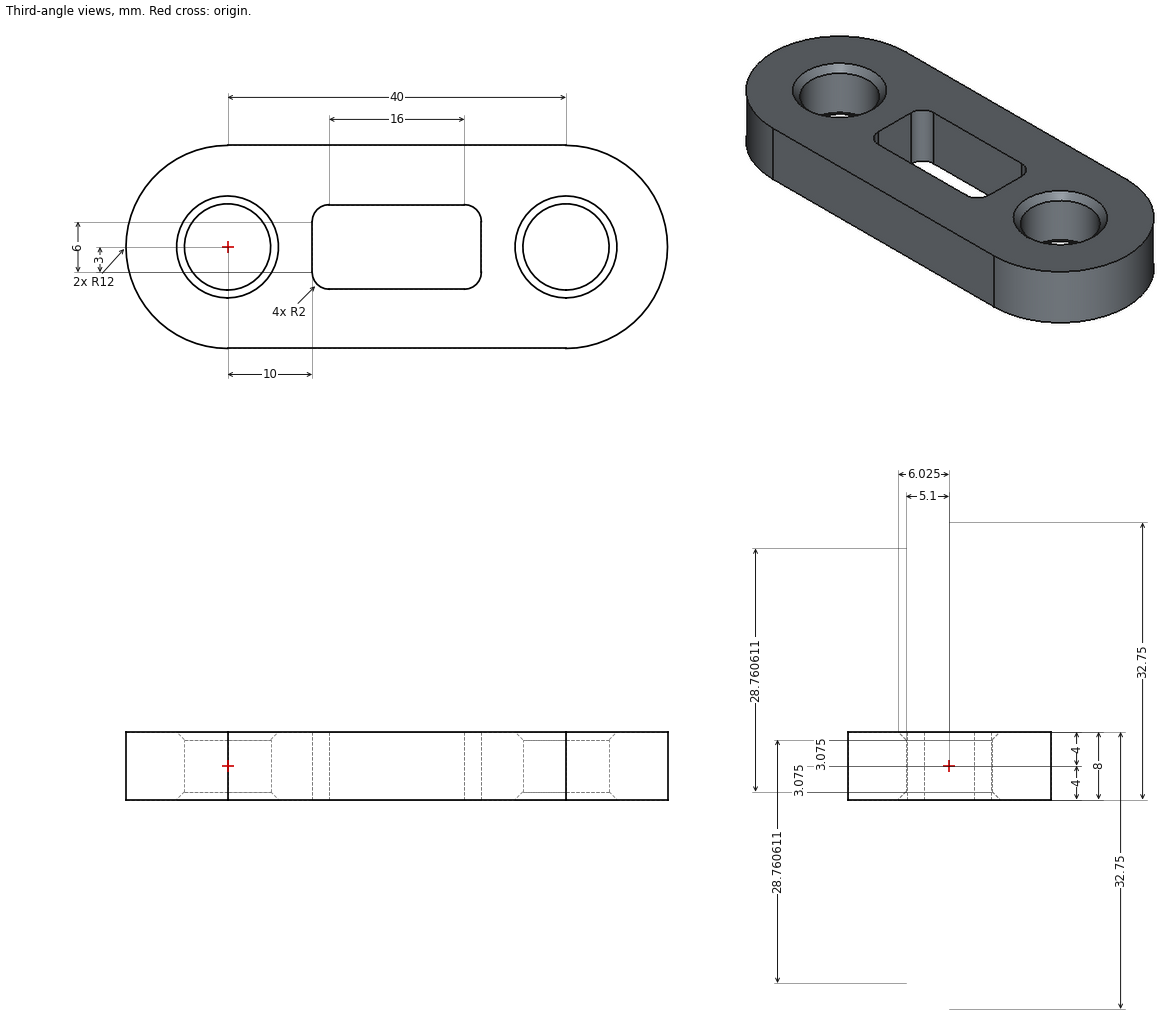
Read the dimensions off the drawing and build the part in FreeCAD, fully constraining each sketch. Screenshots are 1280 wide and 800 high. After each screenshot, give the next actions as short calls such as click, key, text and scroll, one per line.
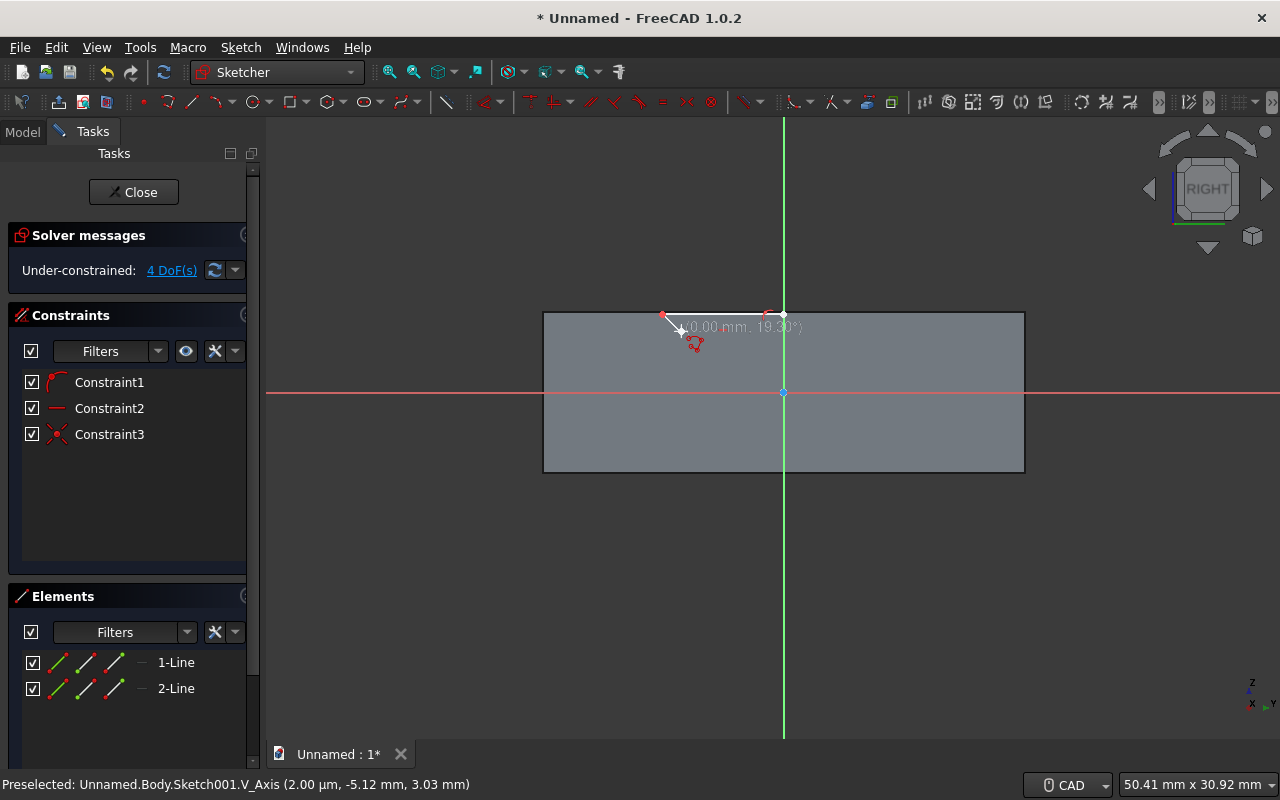
scroll(682, 168, down, 3)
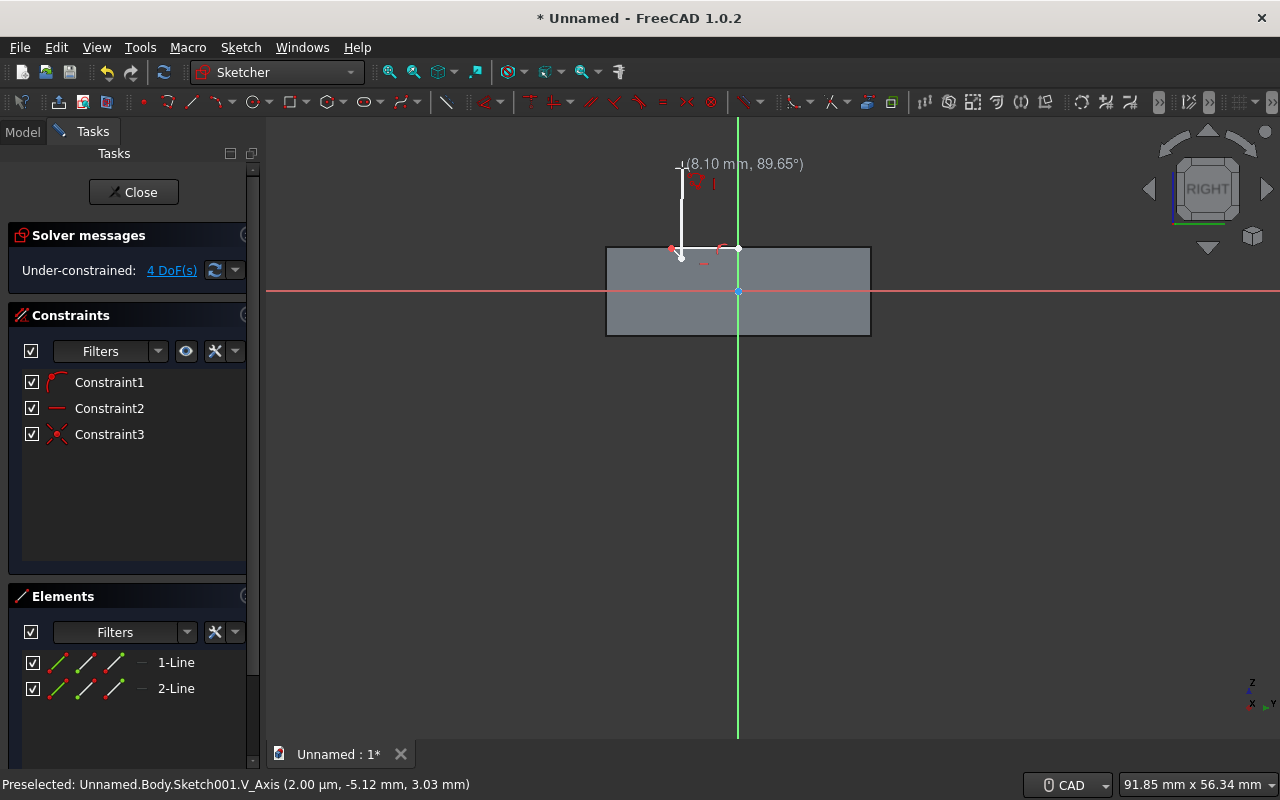
click(682, 575)
click(729, 609)
click(738, 248)
key(Escape)
key(Escape)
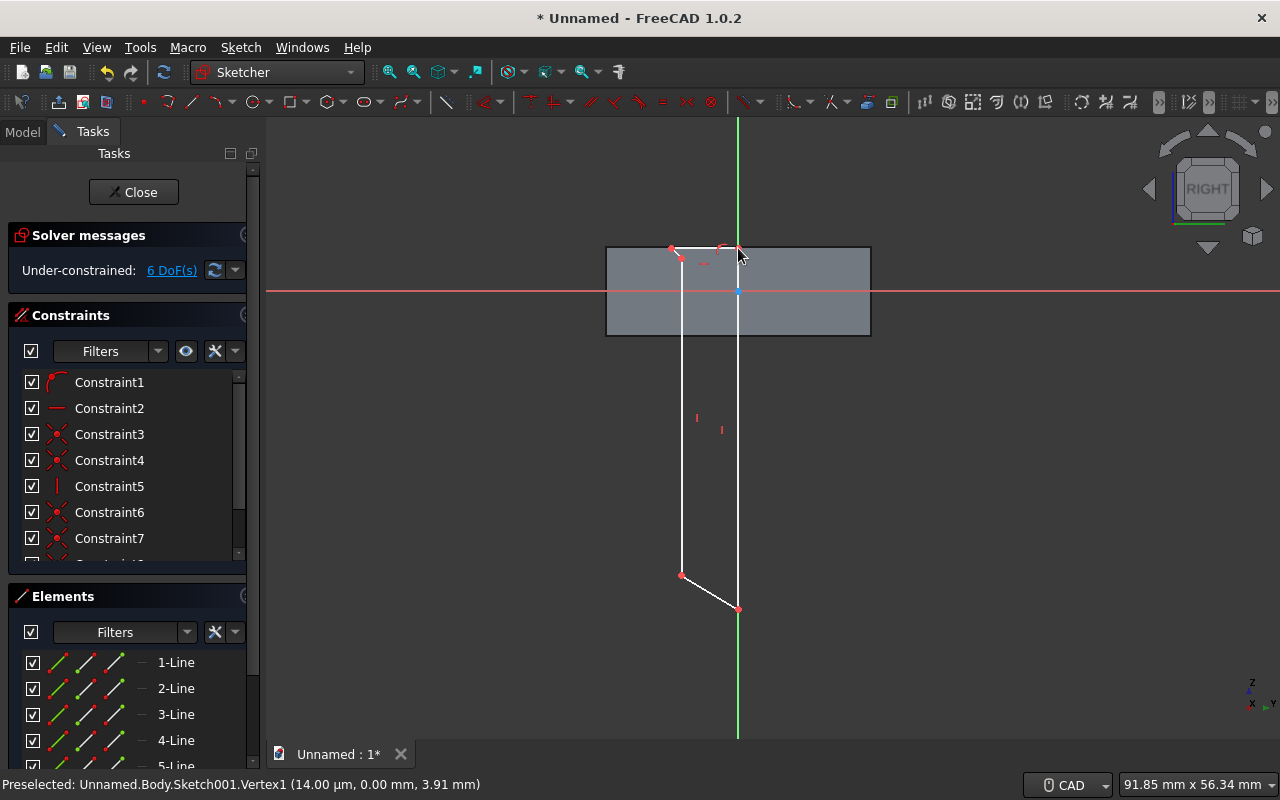
click(484, 102)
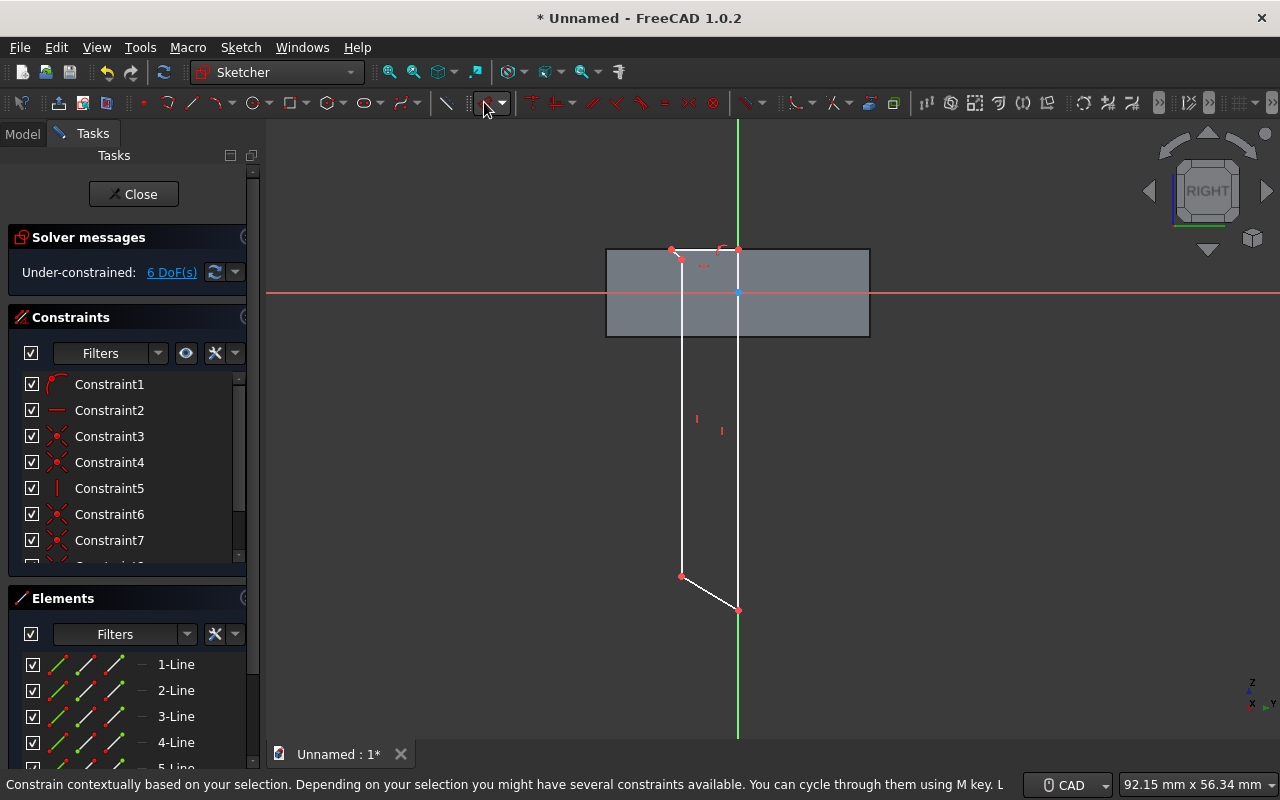
click(738, 250)
click(772, 271)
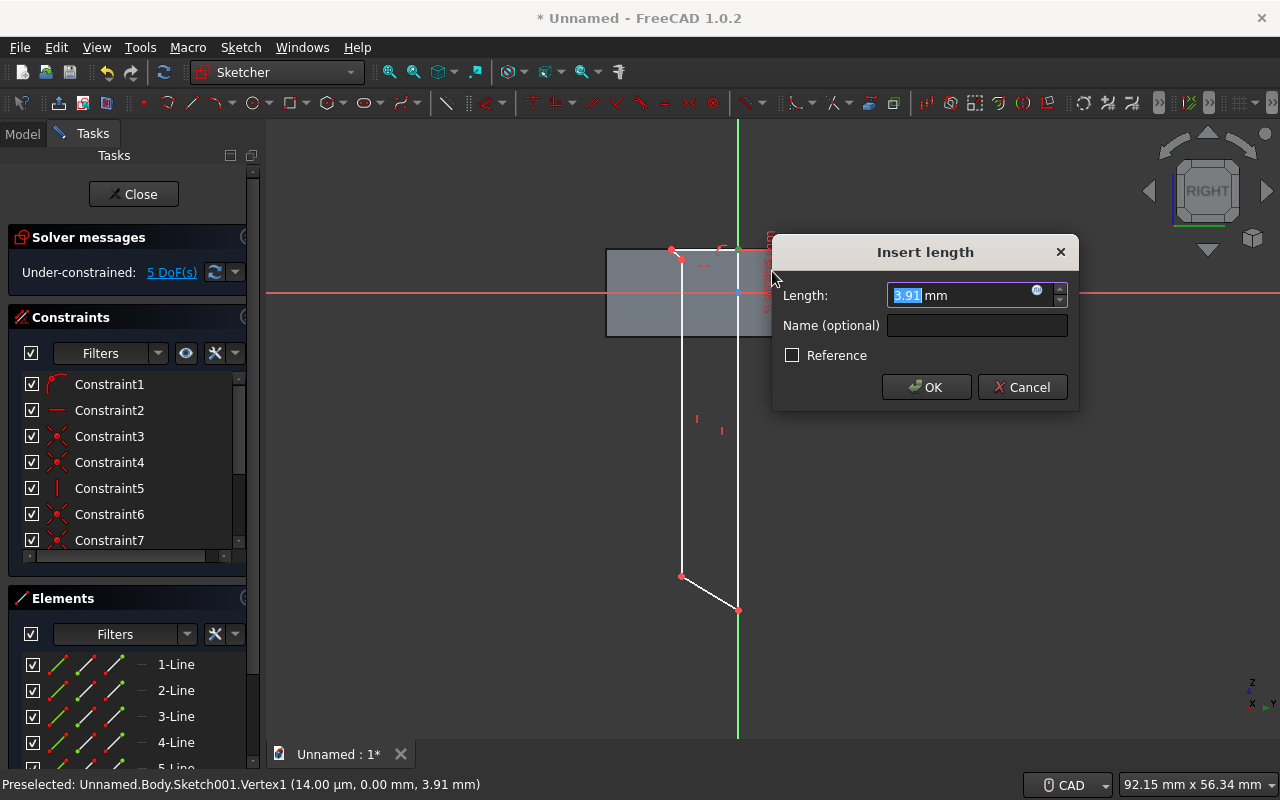
text(4)
key(Return)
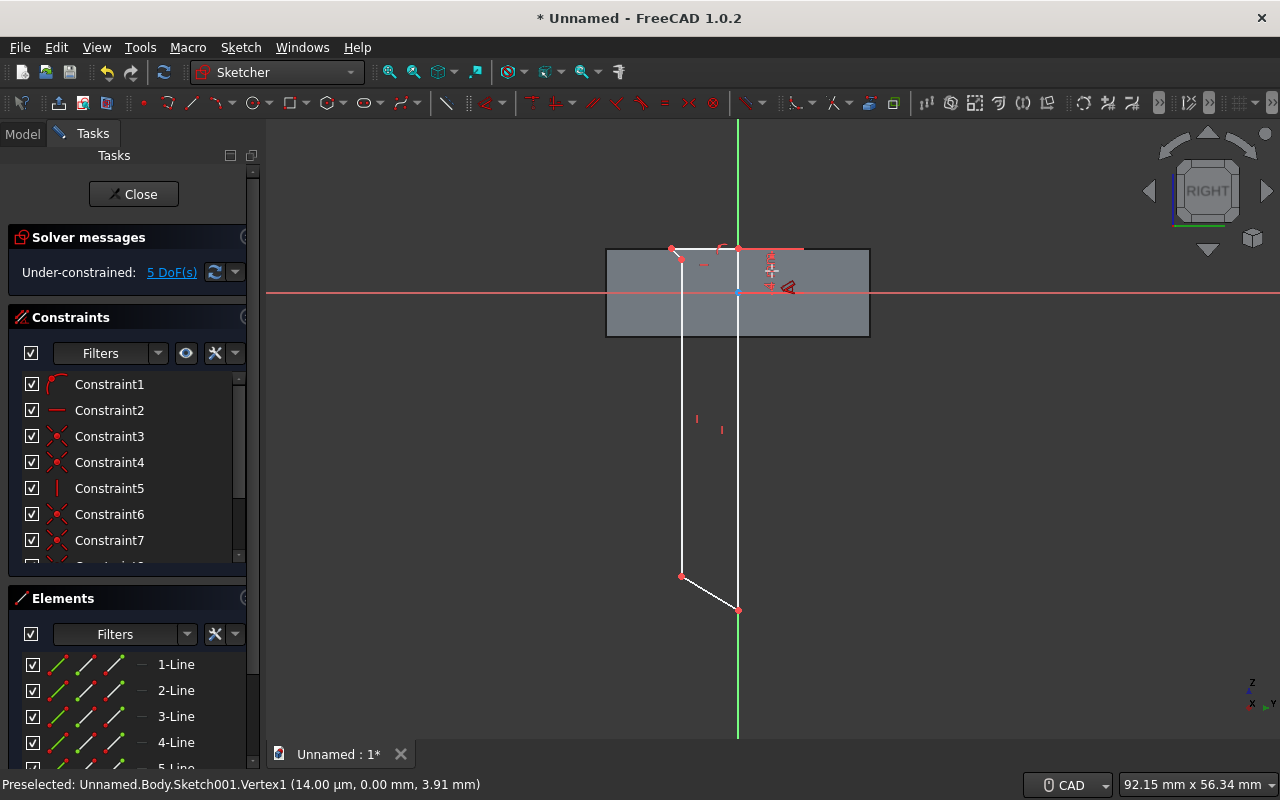
click(682, 260)
click(710, 226)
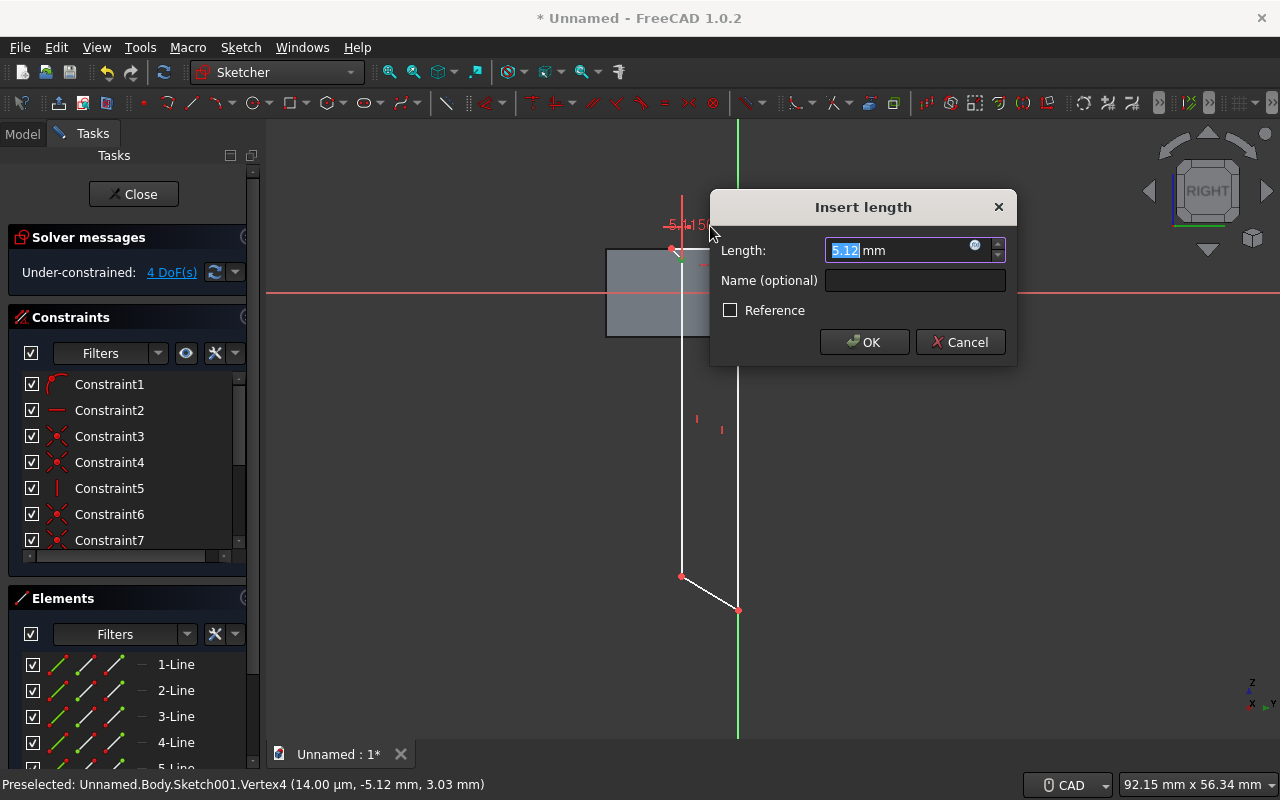
text(5.1)
key(Return)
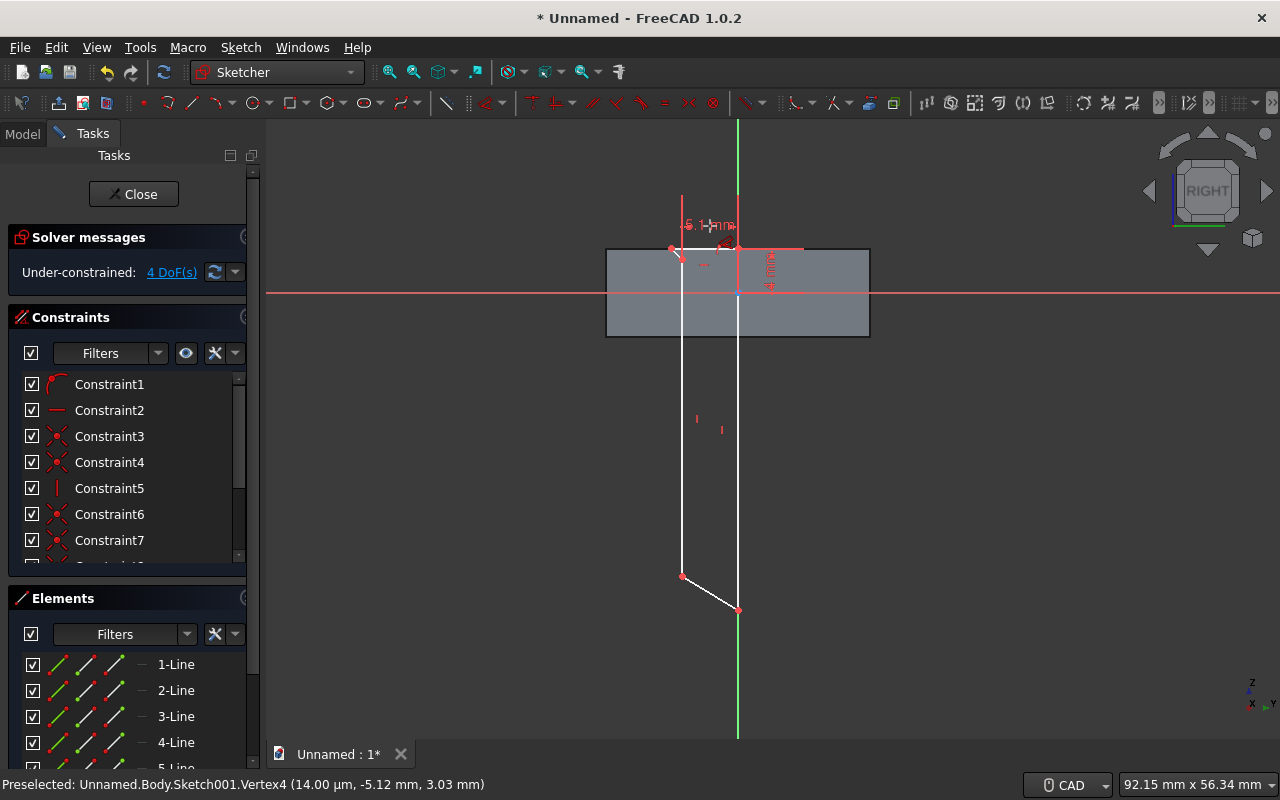
click(718, 249)
click(705, 191)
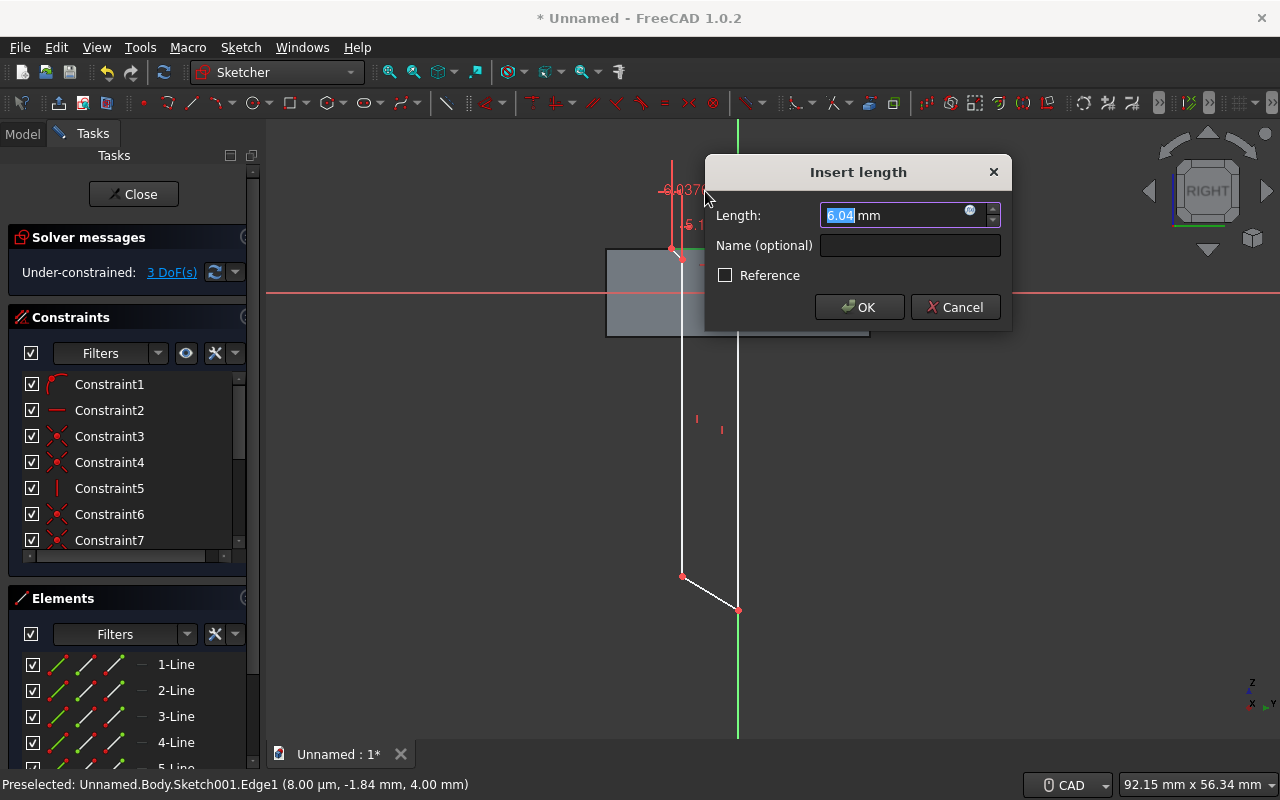
text(6.025)
key(Return)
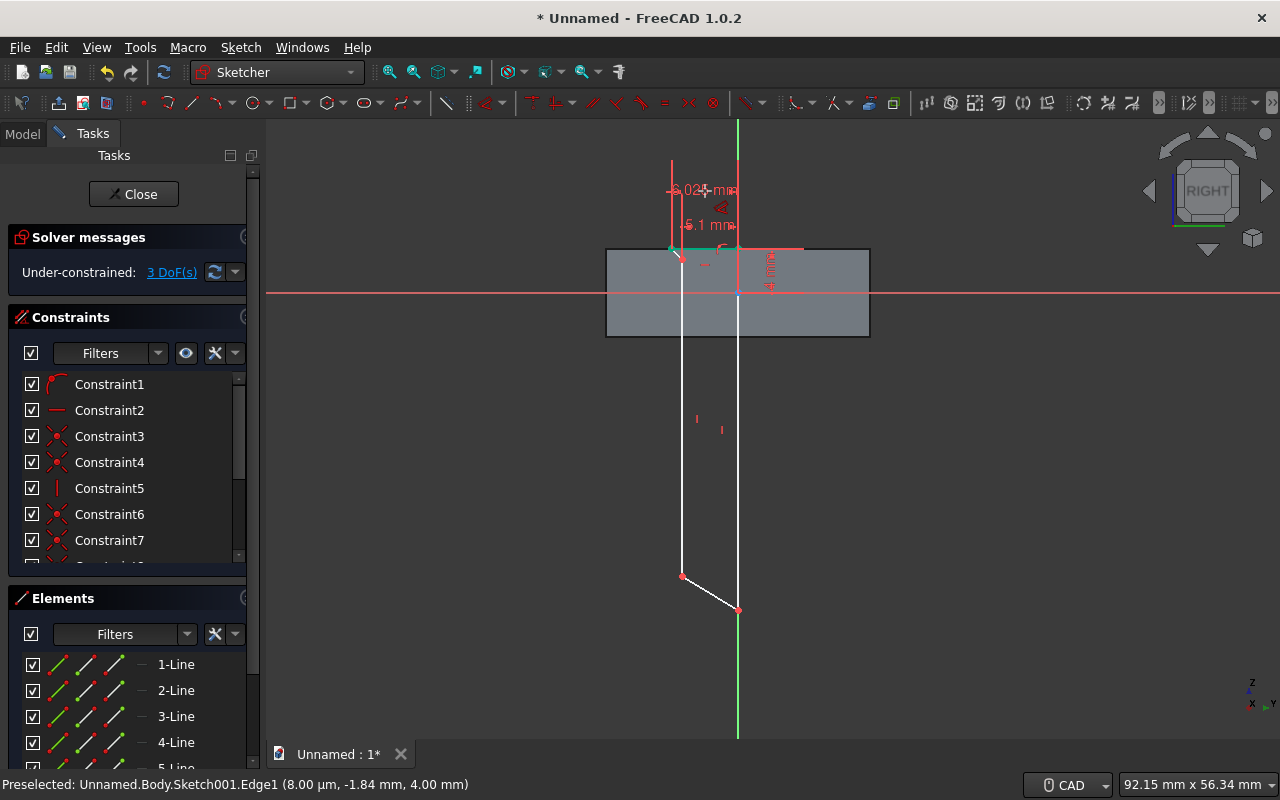
click(738, 502)
click(772, 430)